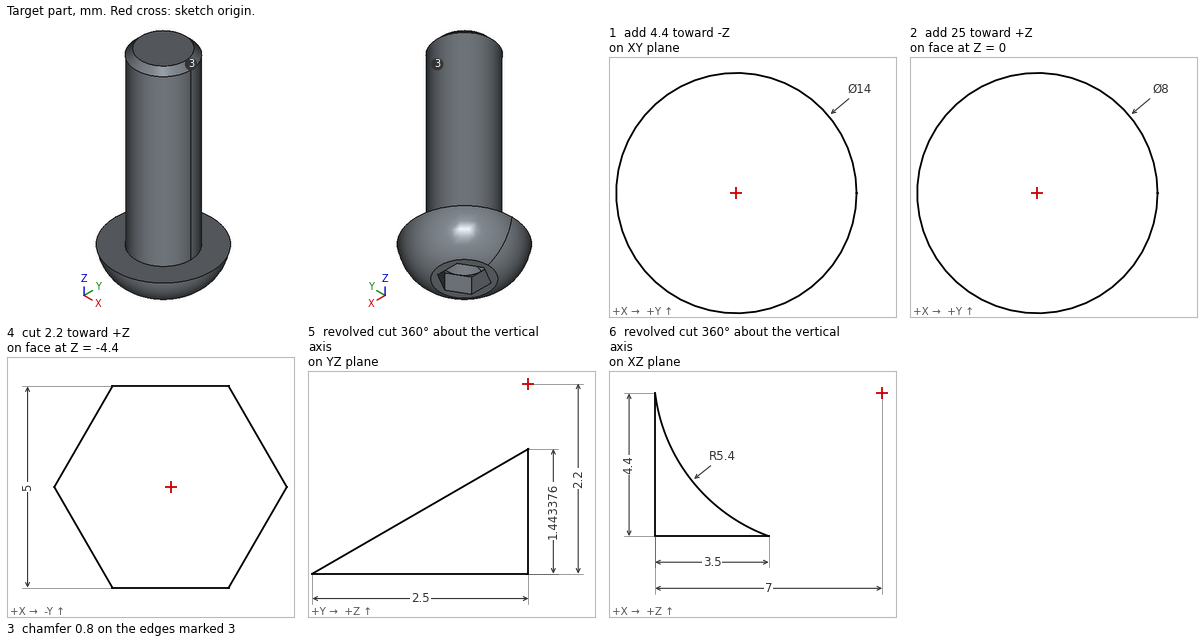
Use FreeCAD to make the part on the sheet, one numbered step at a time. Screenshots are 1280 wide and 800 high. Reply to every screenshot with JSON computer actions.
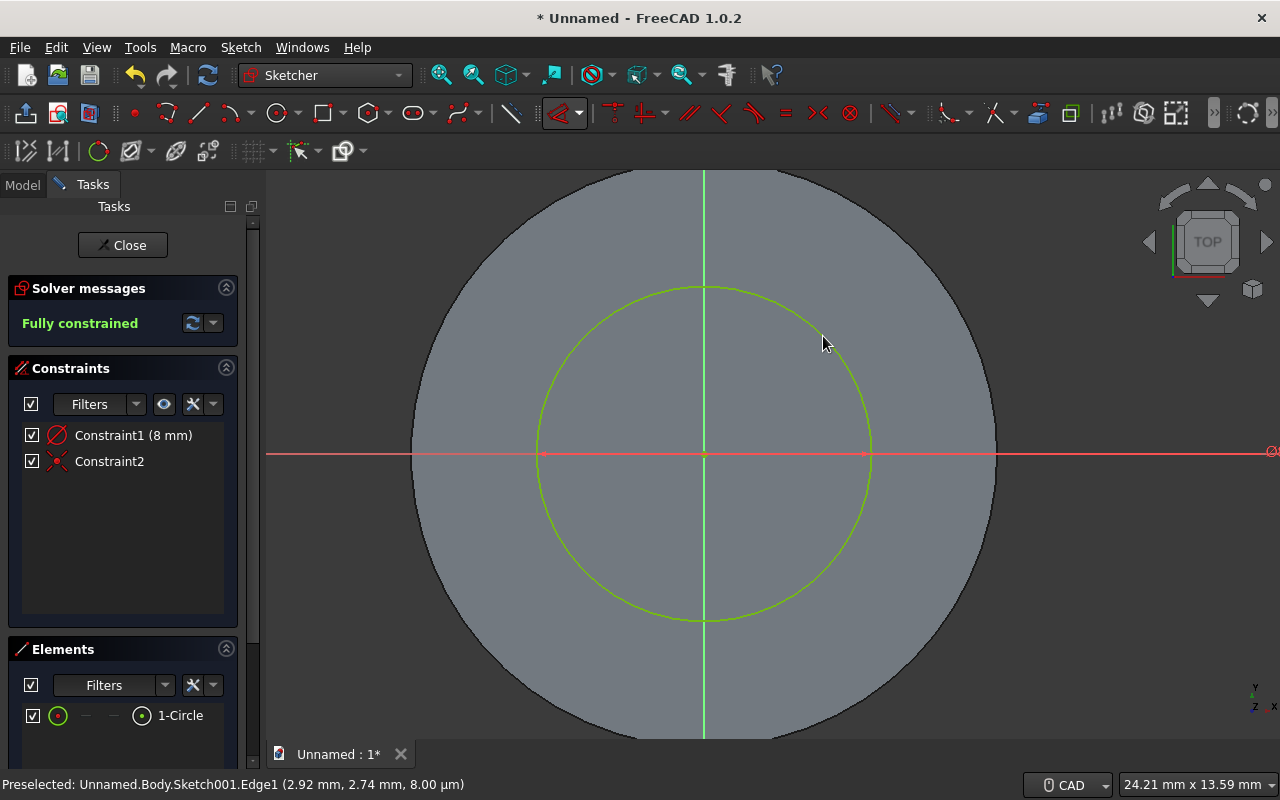
{"action": "left_click", "coordinate": [123, 245]}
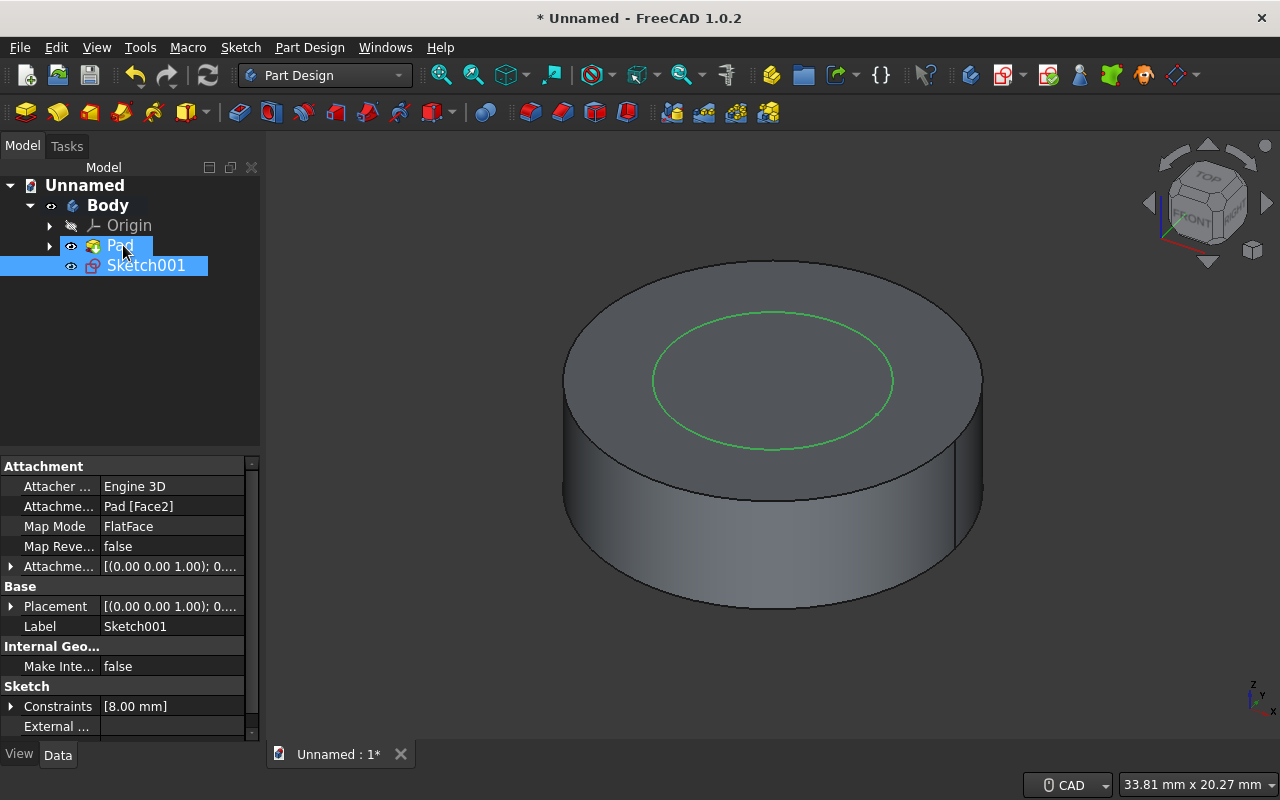
{"action": "left_click", "coordinate": [26, 112]}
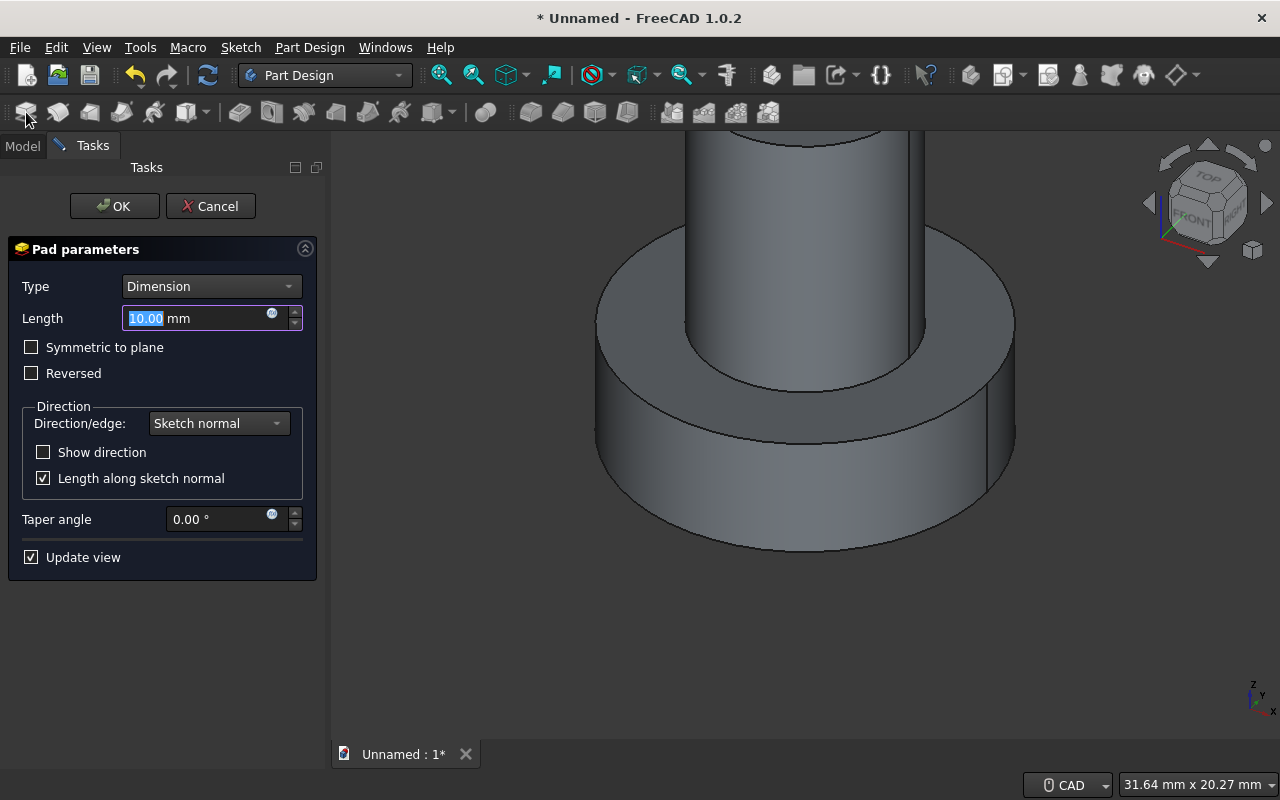
{"action": "type", "text": "25"}
{"action": "key", "text": "Tab"}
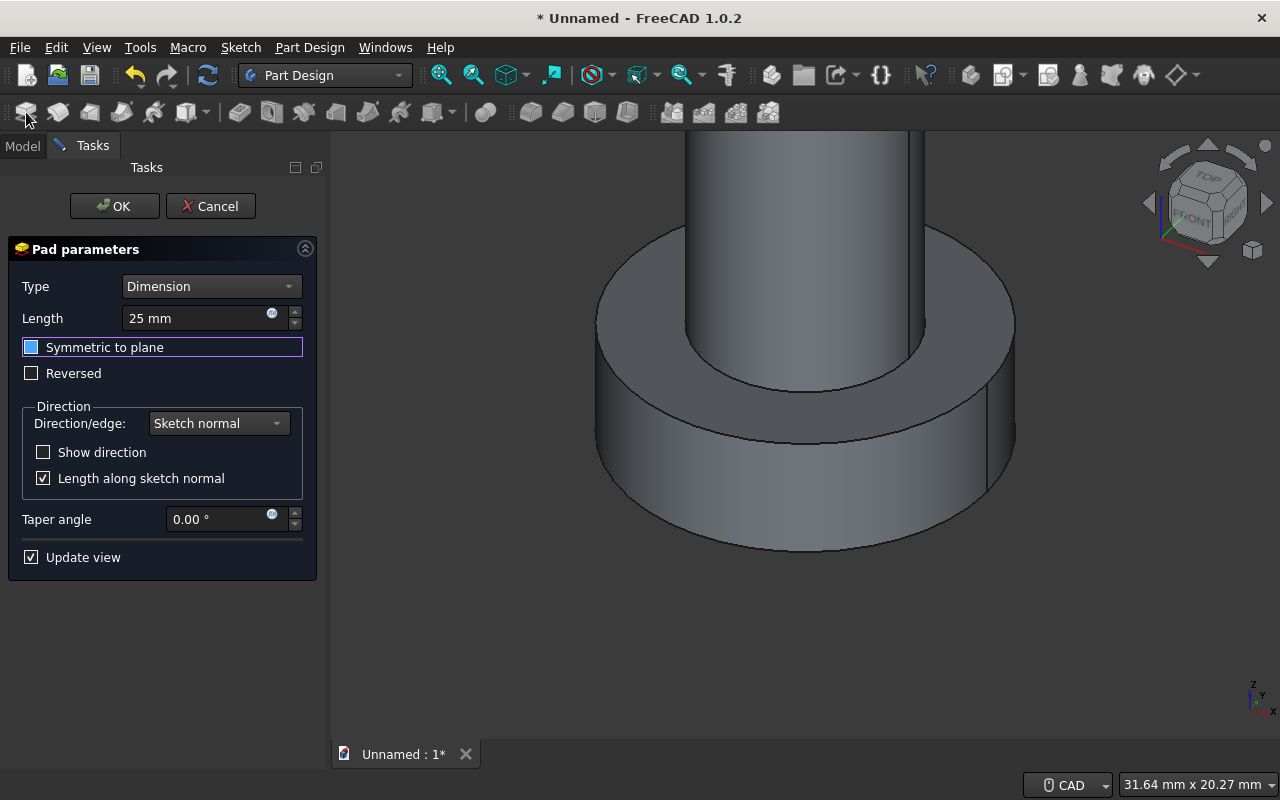
{"action": "left_click", "coordinate": [115, 206]}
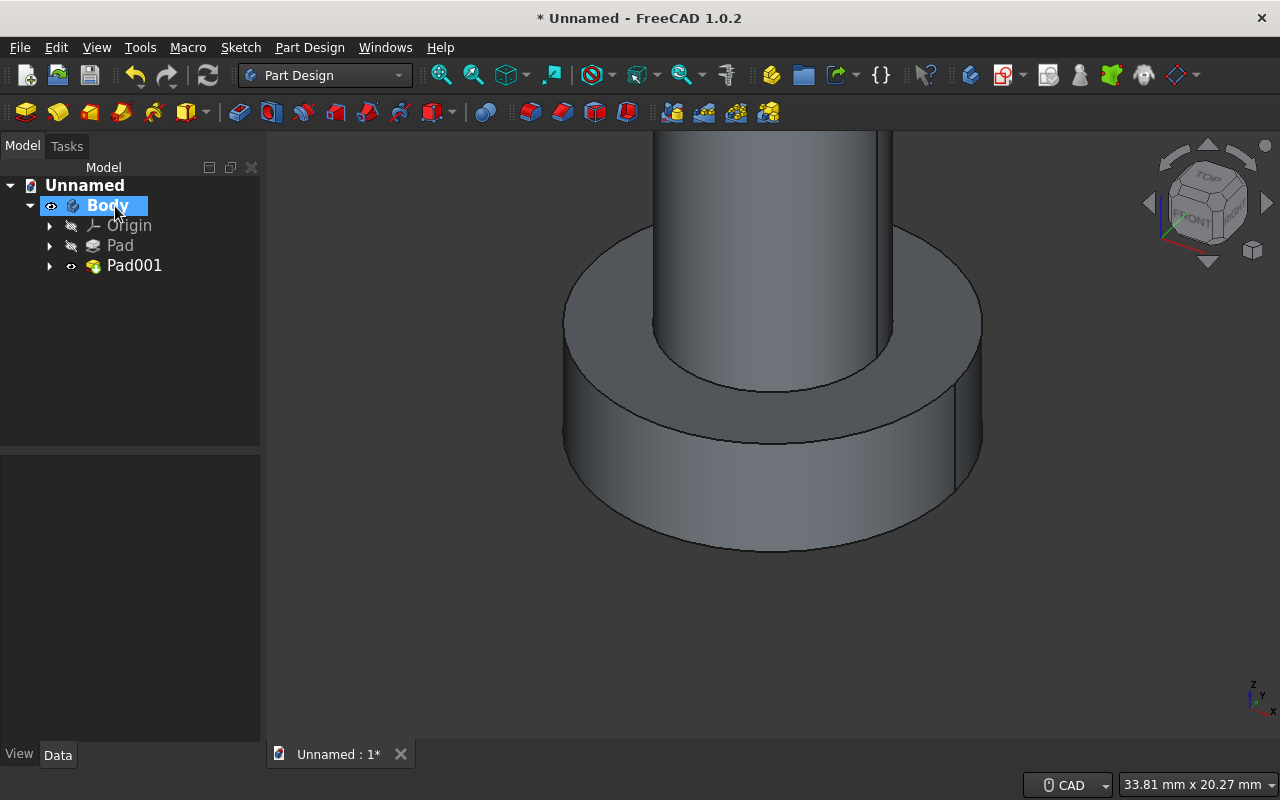
{"action": "left_click", "coordinate": [442, 76]}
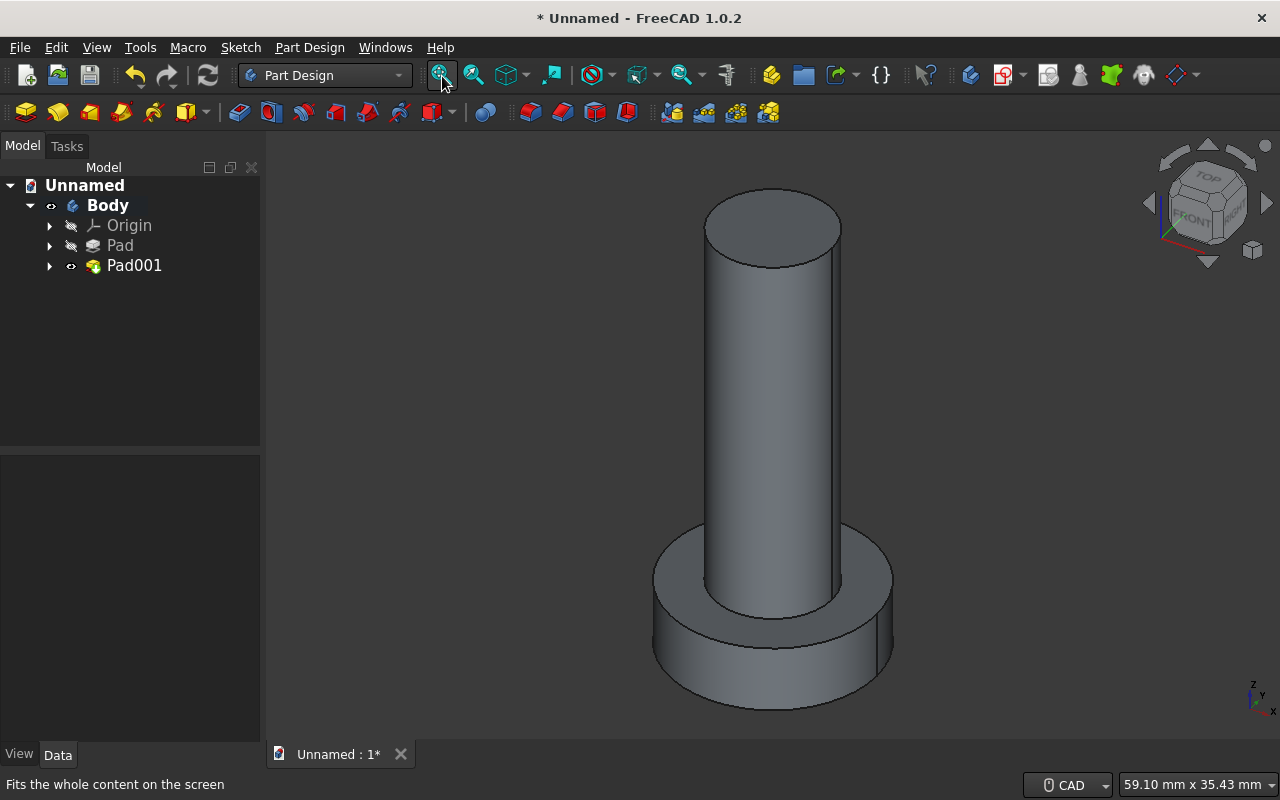
{"action": "left_click", "coordinate": [705, 231]}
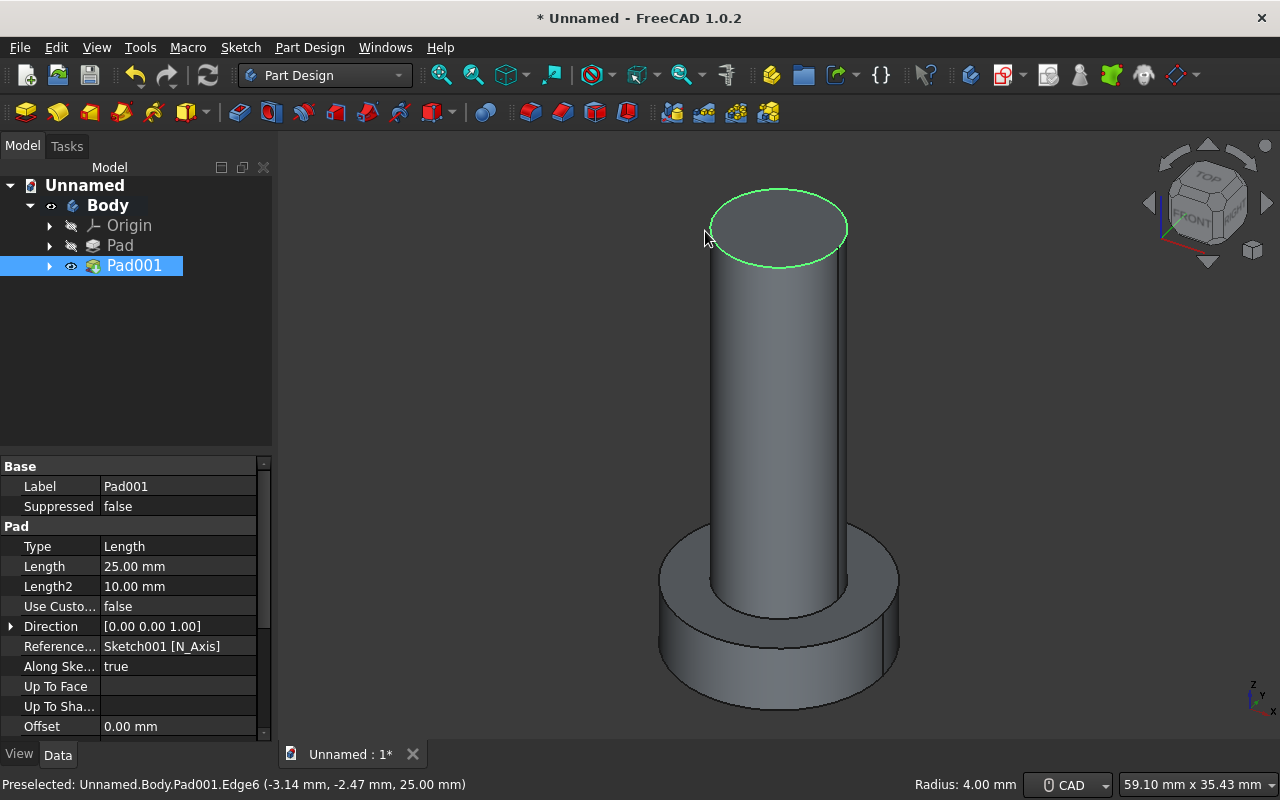
{"action": "left_click", "coordinate": [564, 112]}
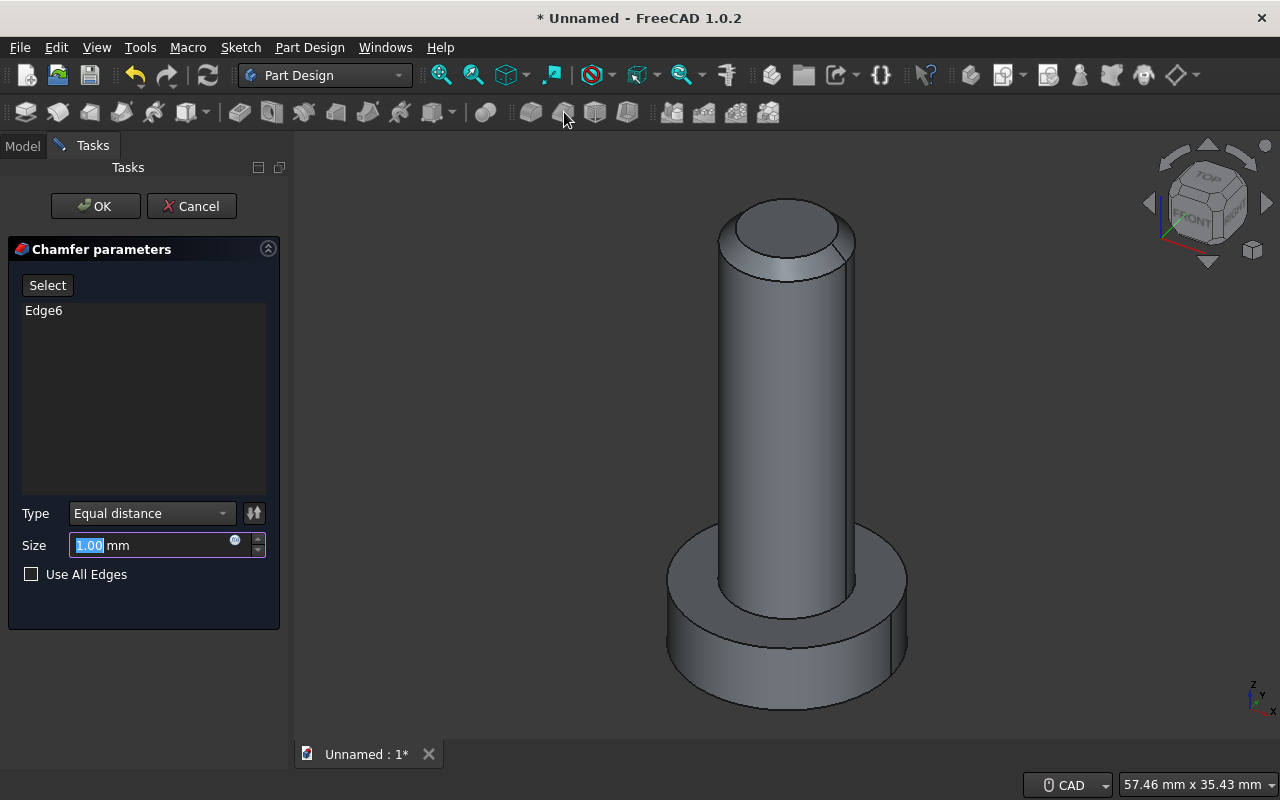
{"action": "type", "text": "0.8"}
{"action": "key", "text": "Tab"}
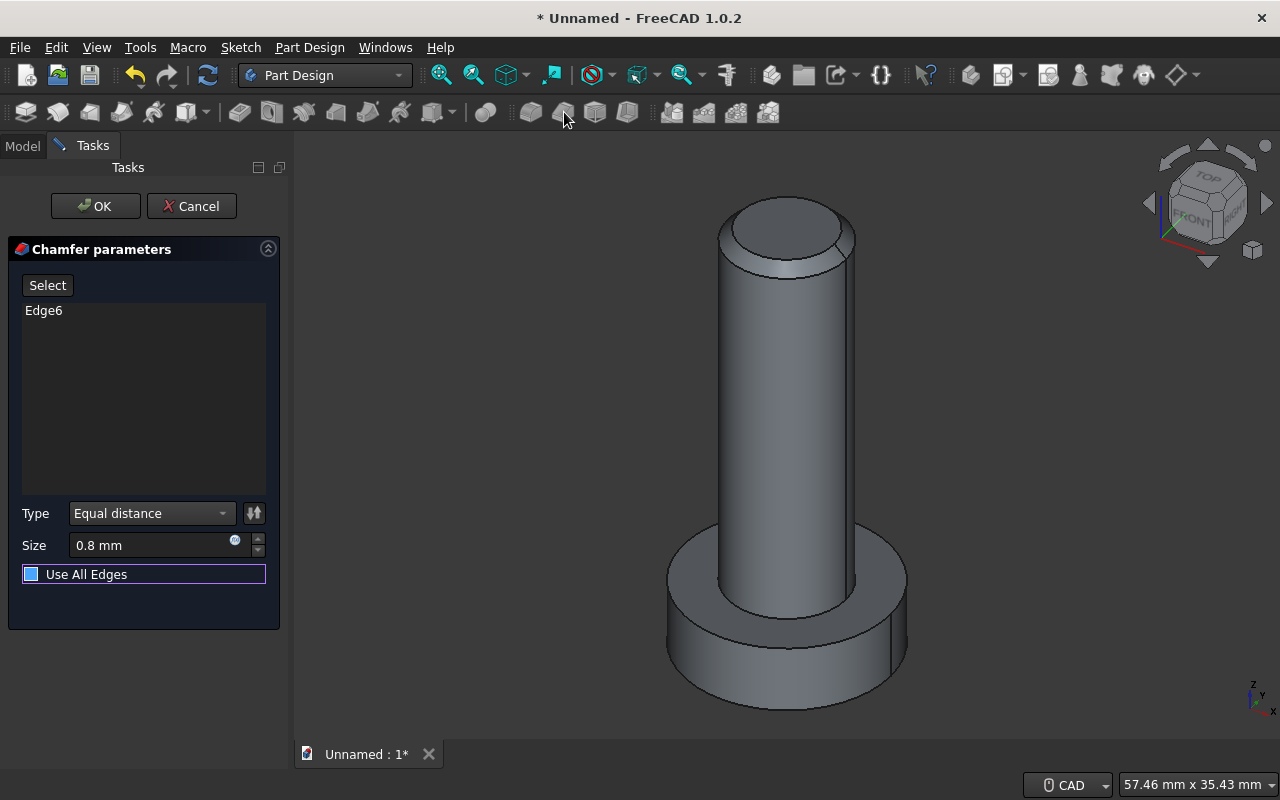
{"action": "left_click", "coordinate": [96, 206]}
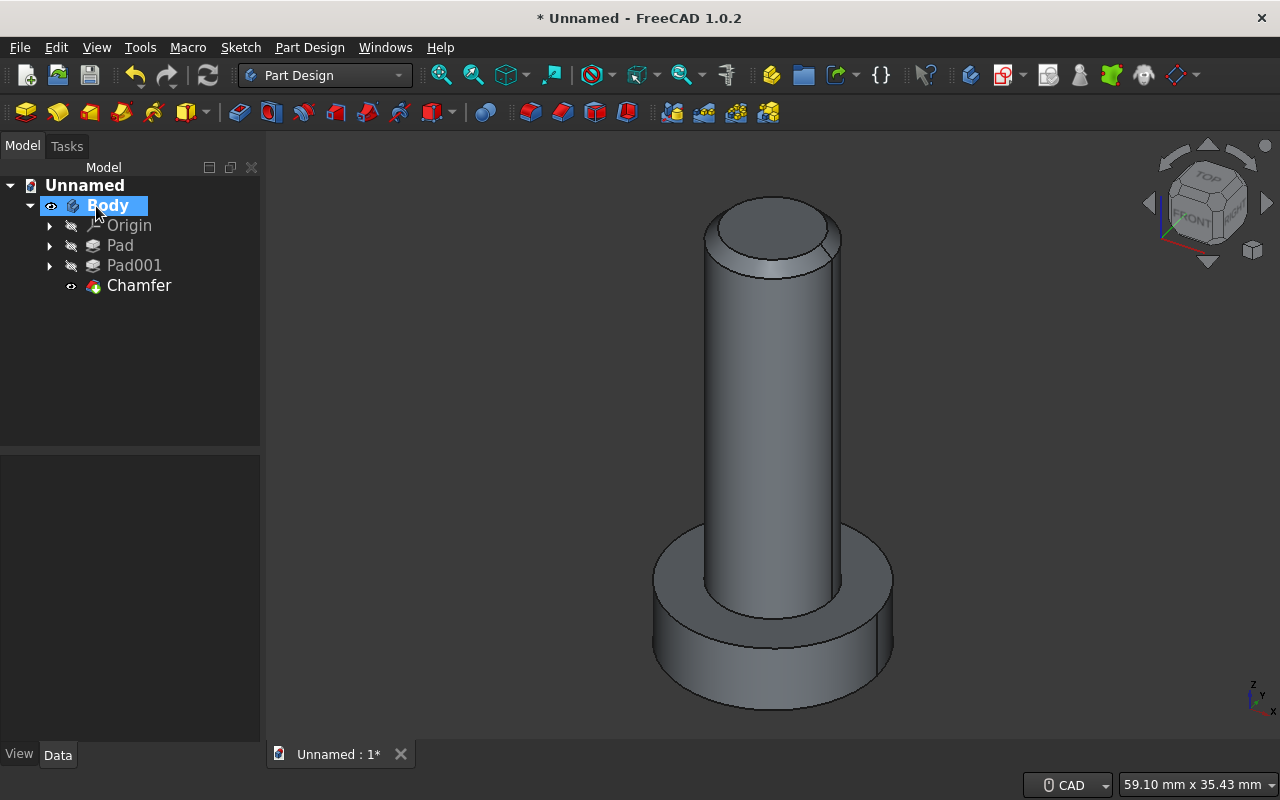
{"action": "key", "text": "5"}